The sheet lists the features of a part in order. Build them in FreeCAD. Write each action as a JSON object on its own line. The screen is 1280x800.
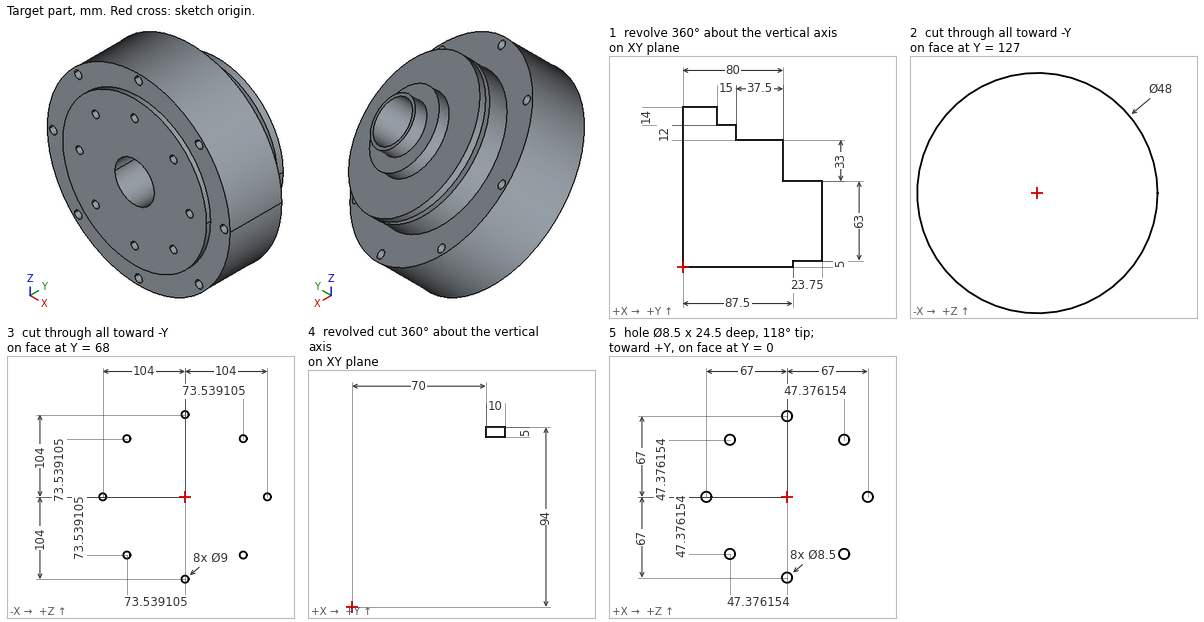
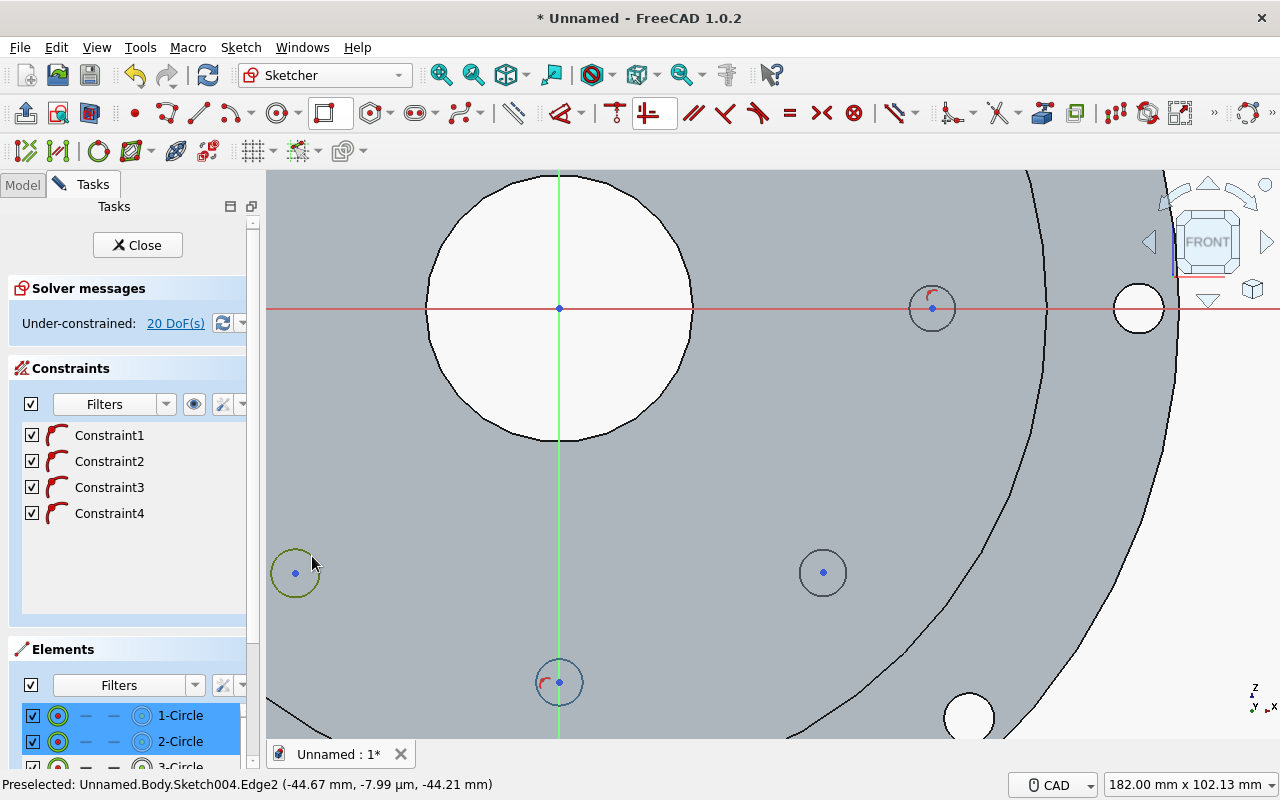
{"action": "scroll", "coordinate": [823, 574], "scroll_direction": "down", "scroll_amount": 4}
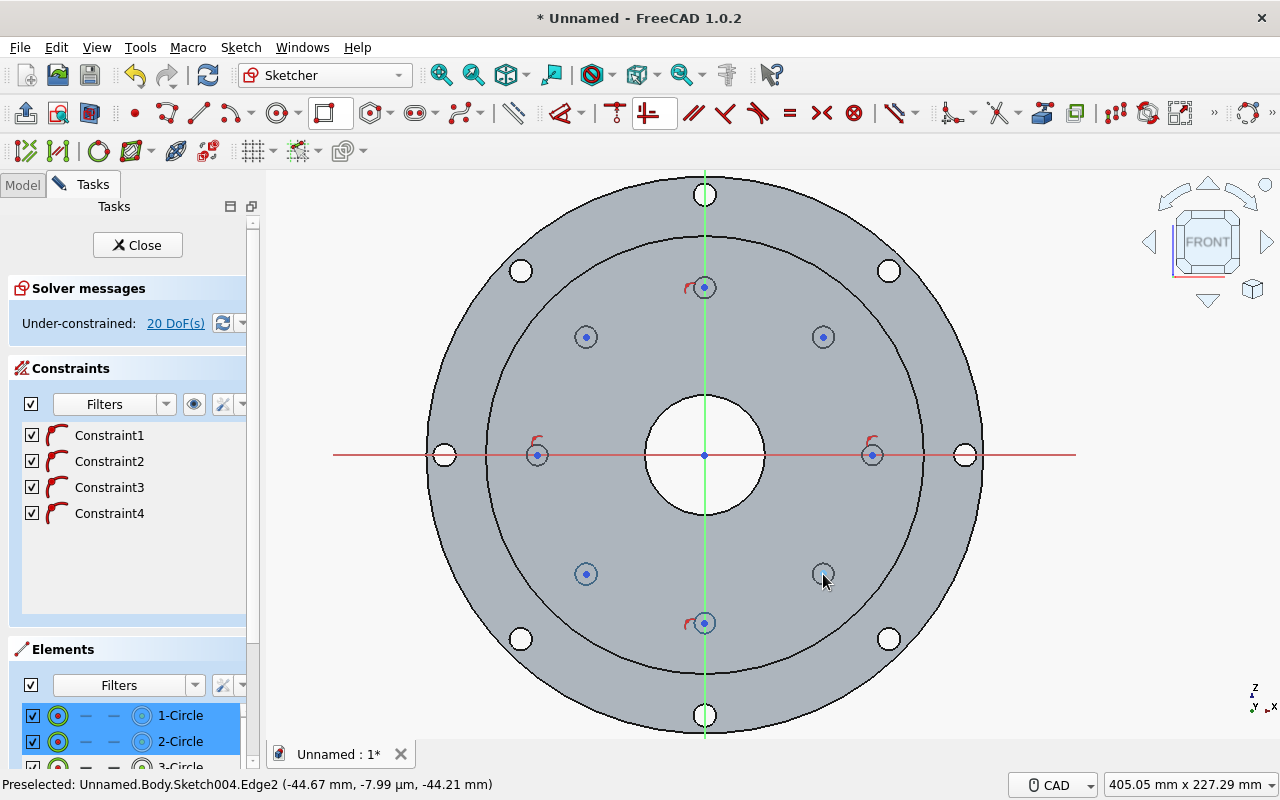
{"action": "scroll", "coordinate": [545, 448], "scroll_direction": "up", "scroll_amount": 4}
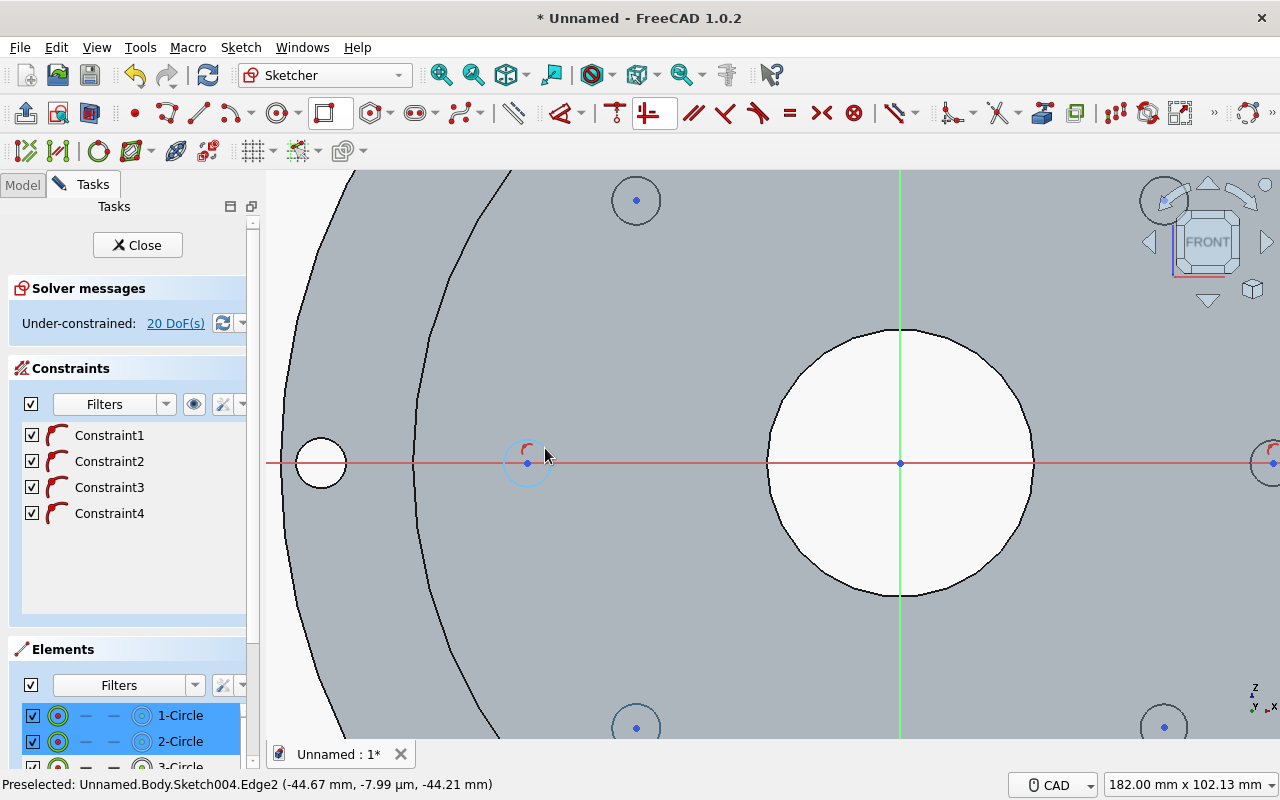
{"action": "left_click", "coordinate": [544, 447]}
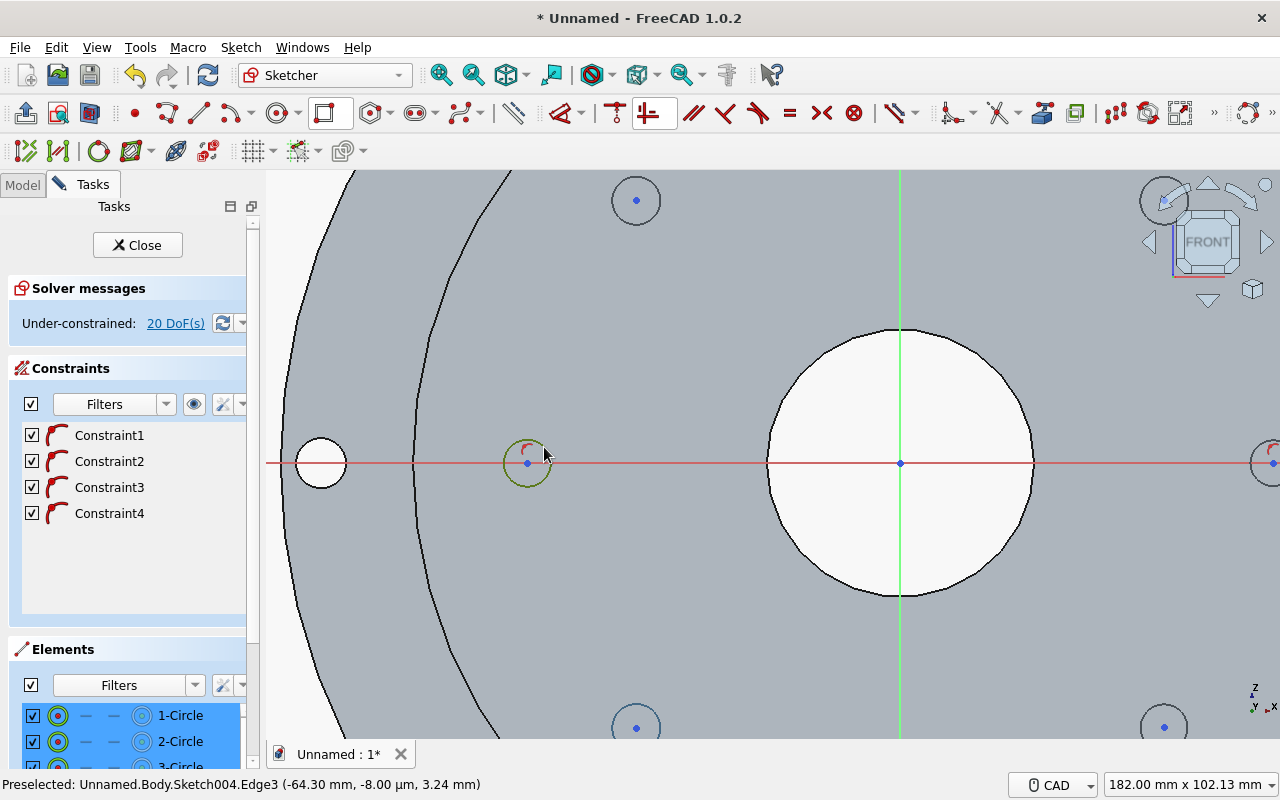
{"action": "left_click", "coordinate": [619, 218]}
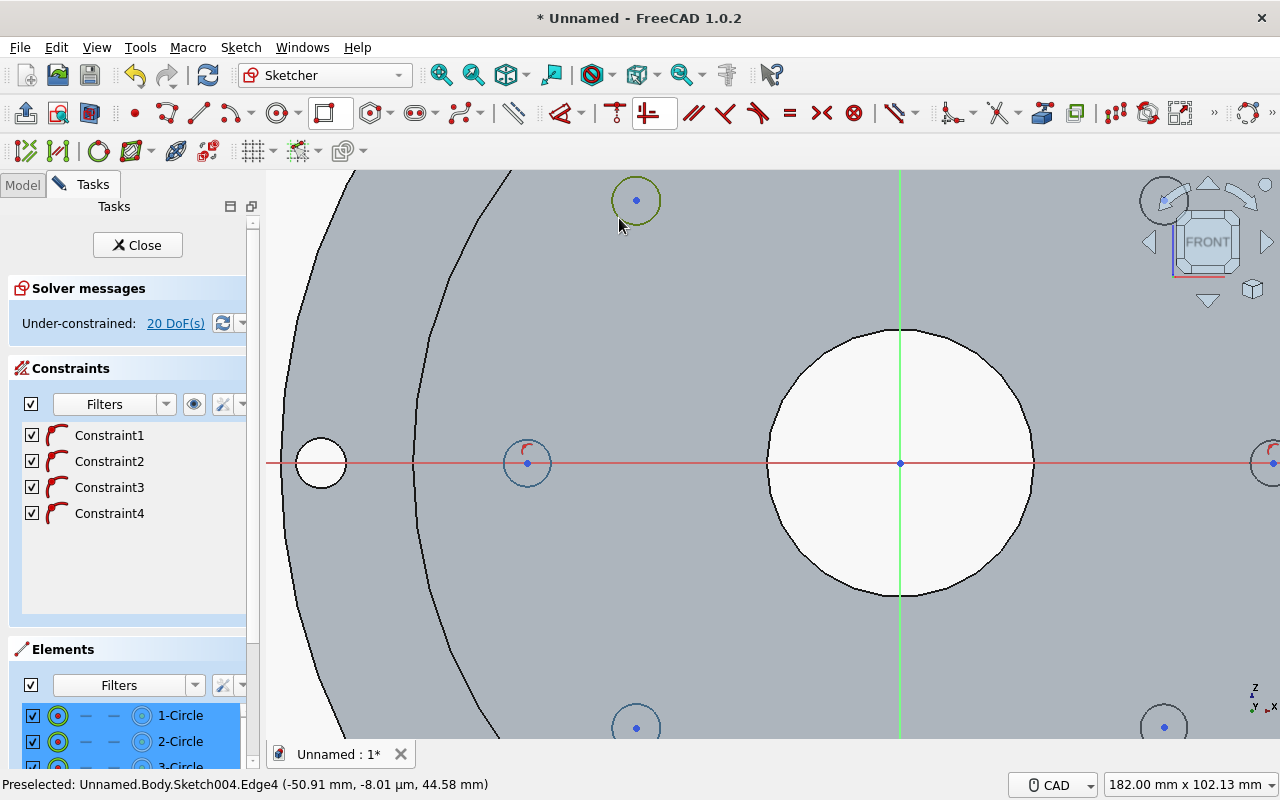
{"action": "scroll", "coordinate": [545, 447], "scroll_direction": "down", "scroll_amount": 4}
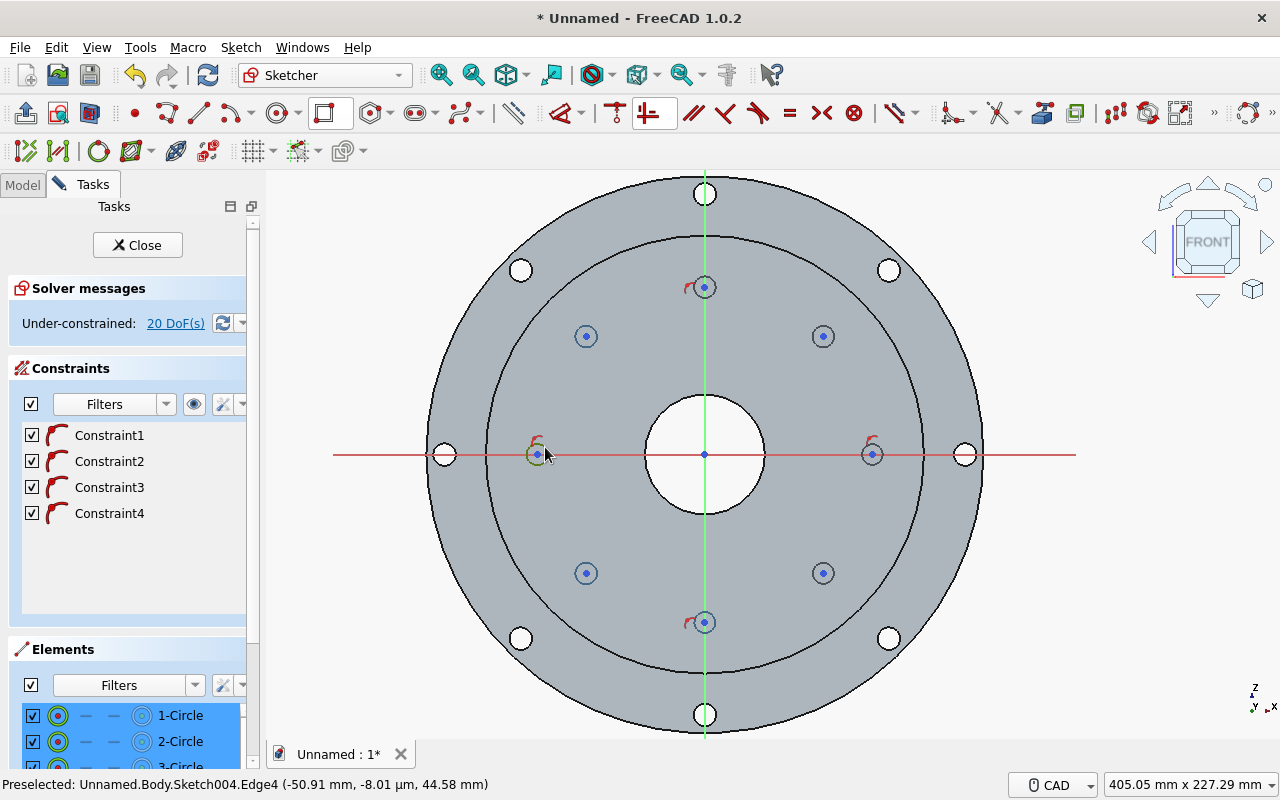
{"action": "scroll", "coordinate": [712, 280], "scroll_direction": "up", "scroll_amount": 4}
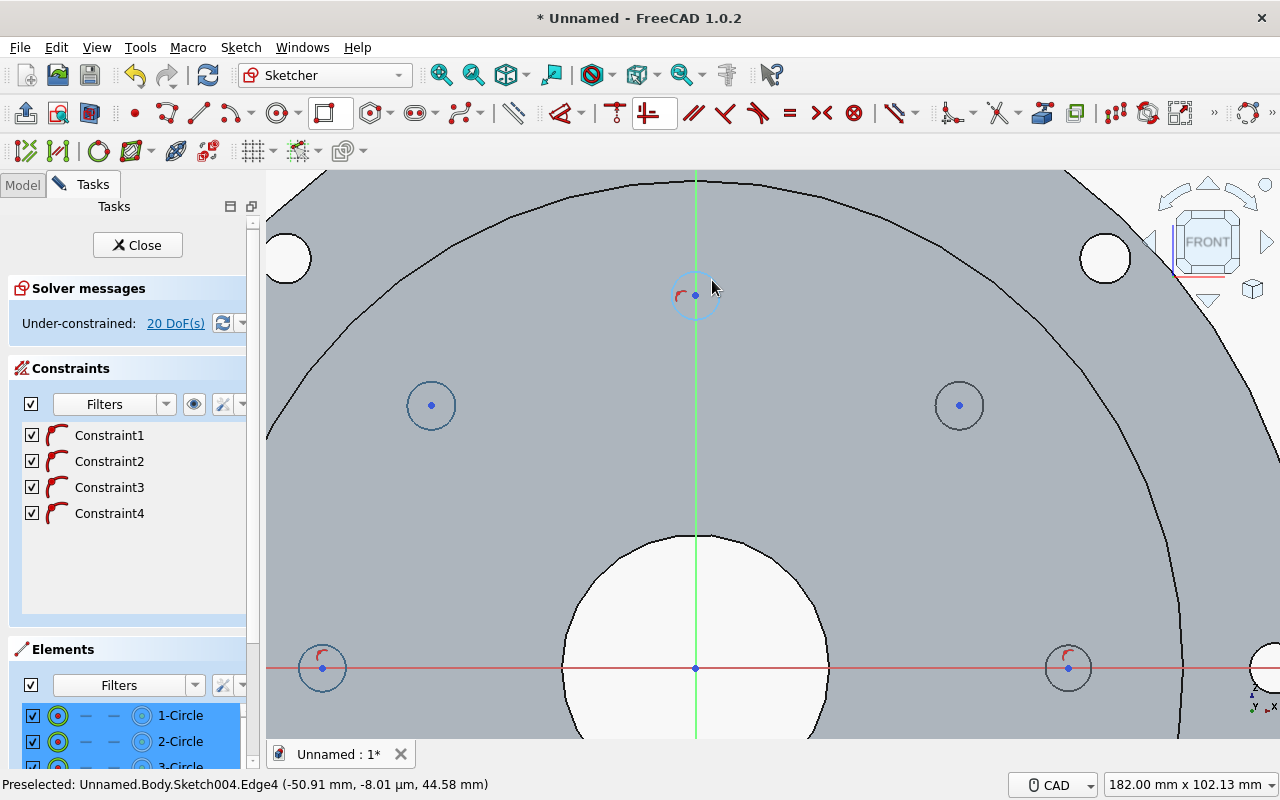
{"action": "left_click", "coordinate": [712, 279]}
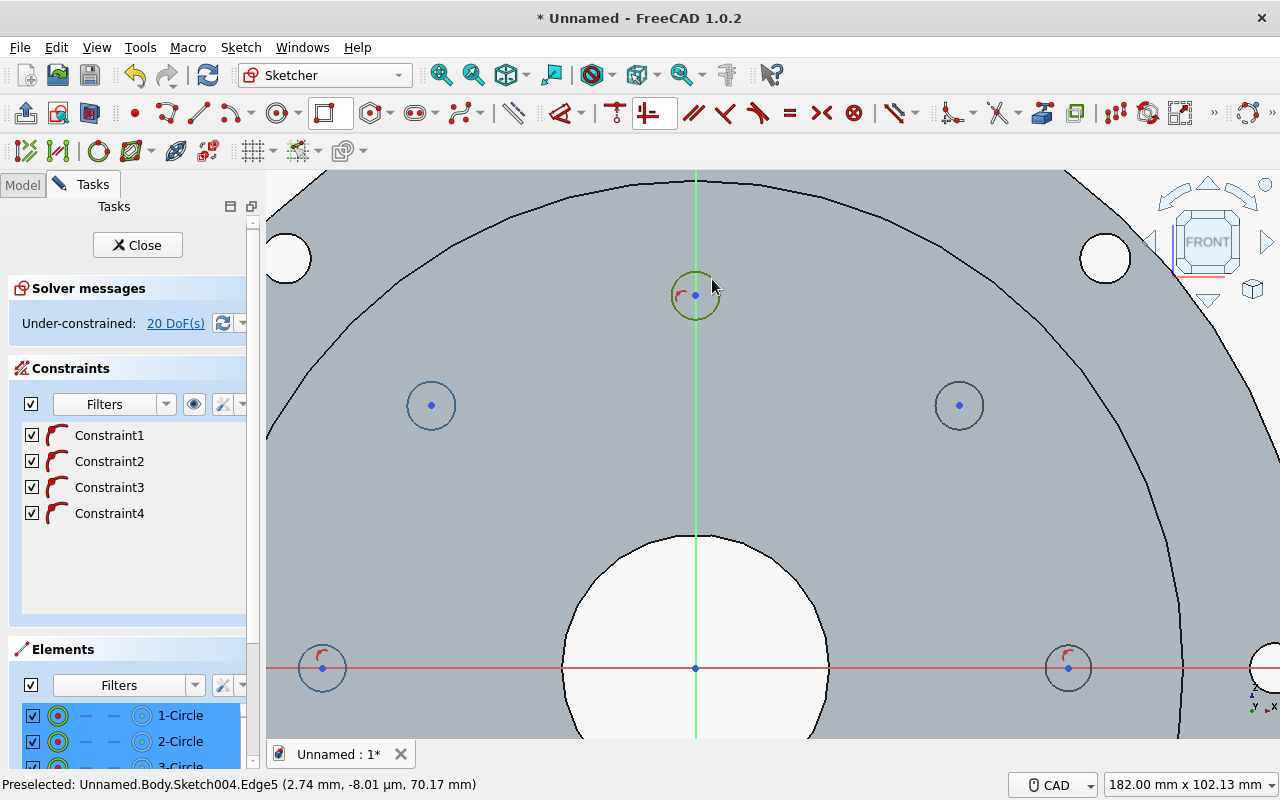
{"action": "left_click", "coordinate": [976, 389]}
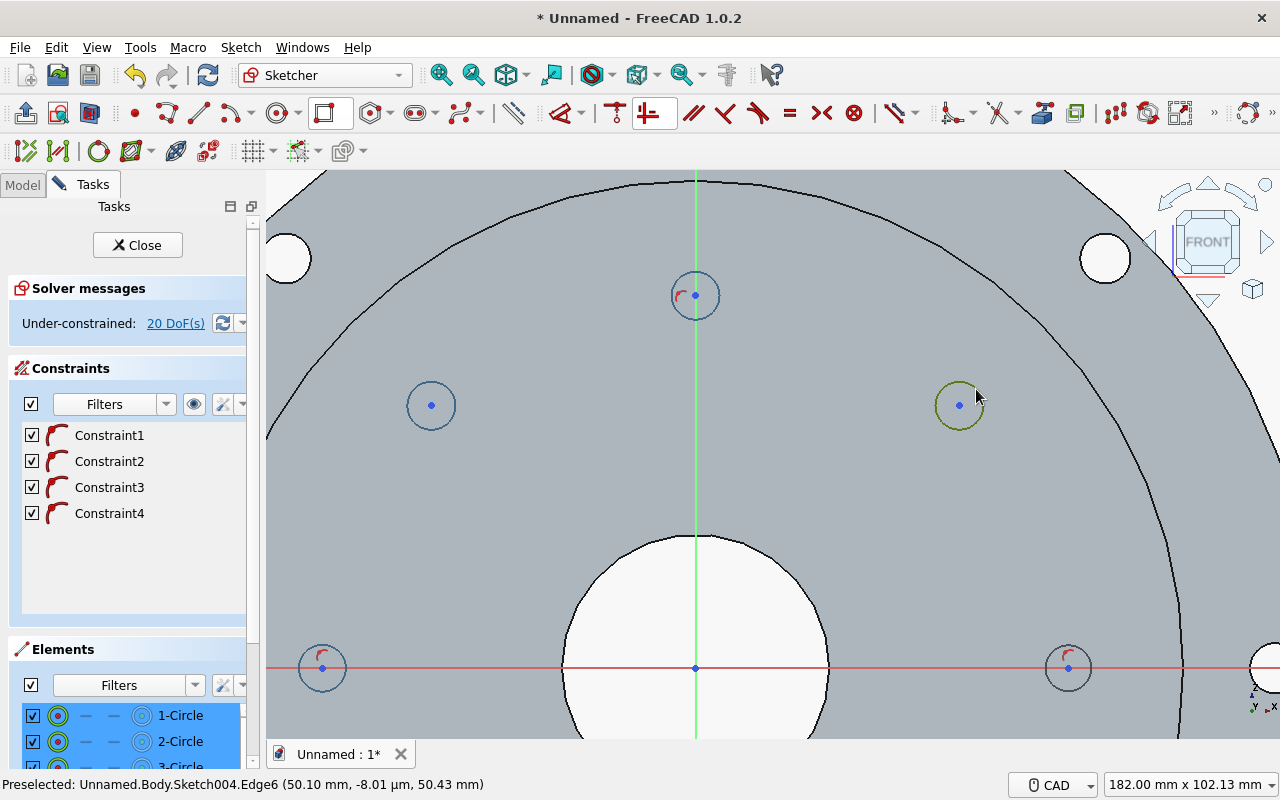
{"action": "left_click", "coordinate": [1085, 652]}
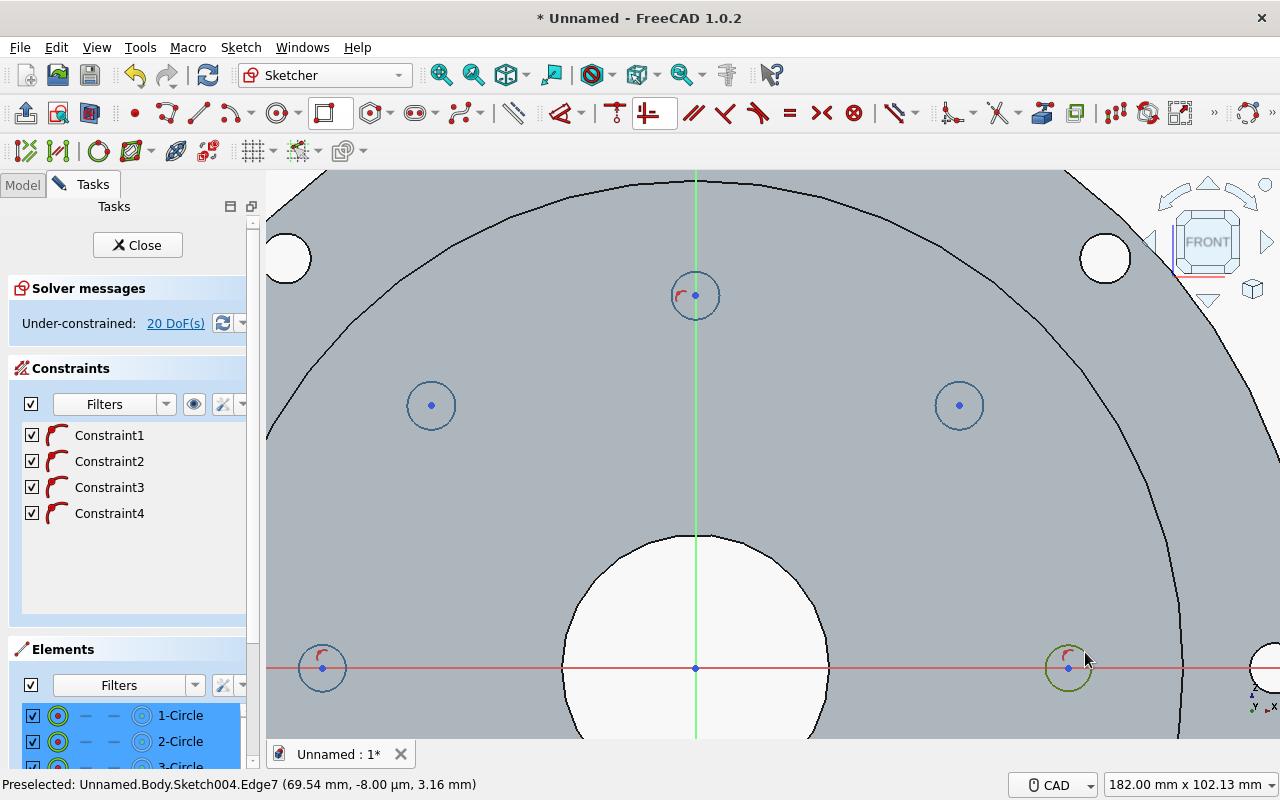
{"action": "scroll", "coordinate": [712, 280], "scroll_direction": "down", "scroll_amount": 4}